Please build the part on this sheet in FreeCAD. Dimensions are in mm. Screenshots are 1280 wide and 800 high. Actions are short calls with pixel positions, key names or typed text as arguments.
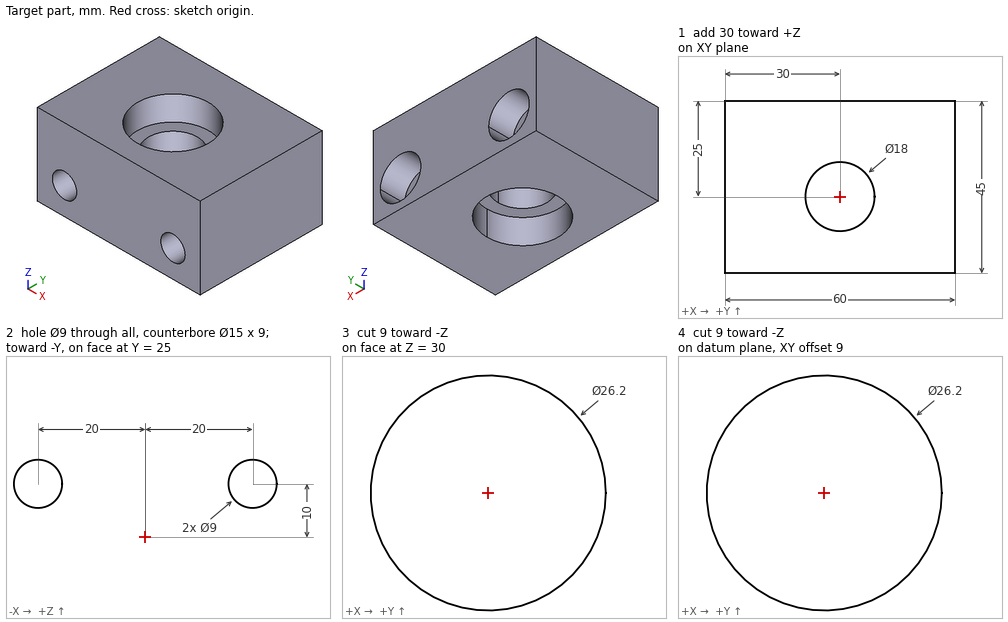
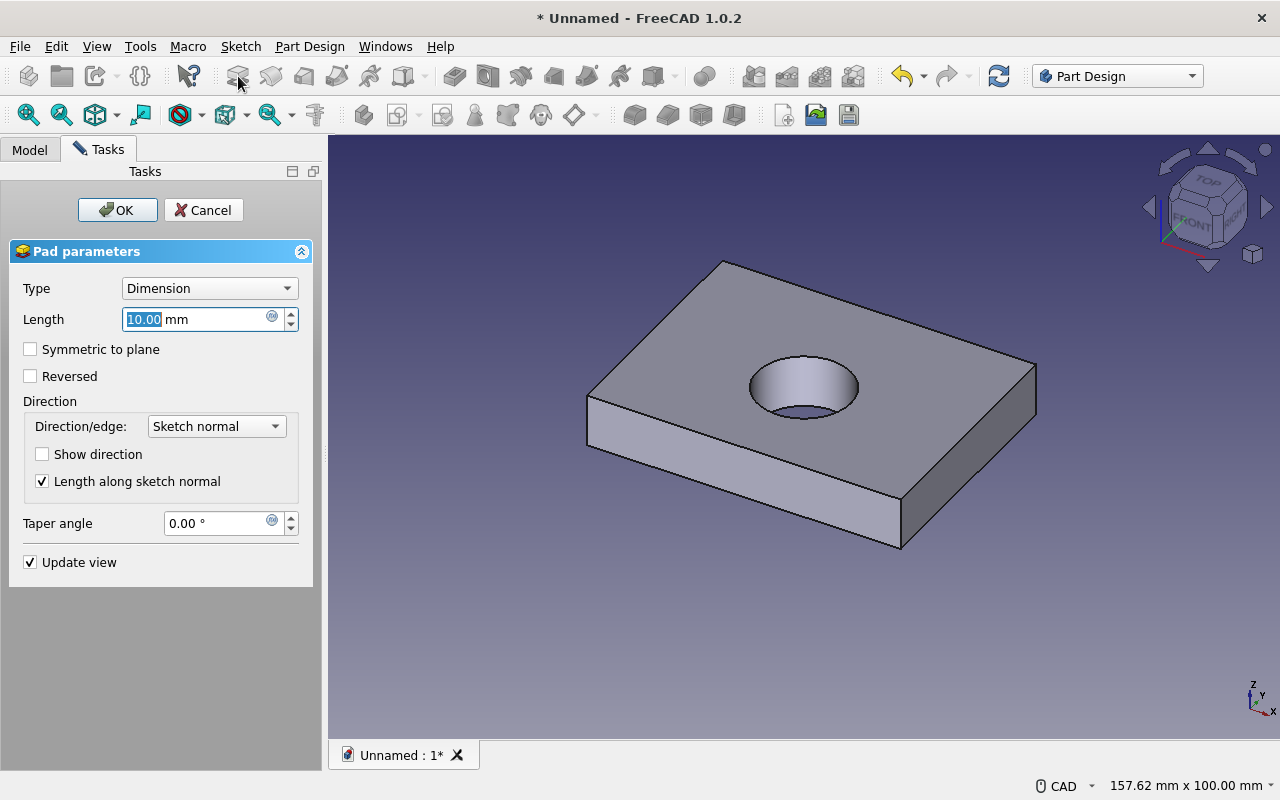
text(30)
key(Tab)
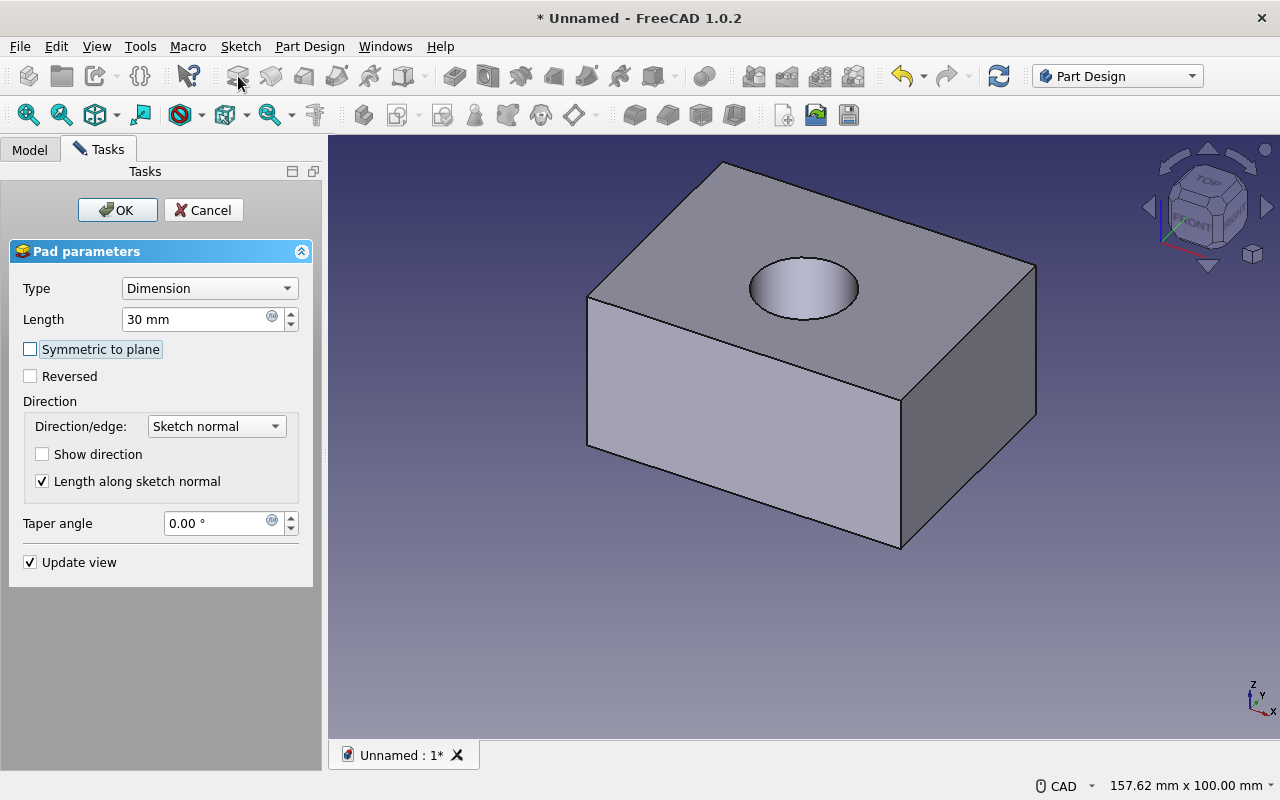
click(118, 210)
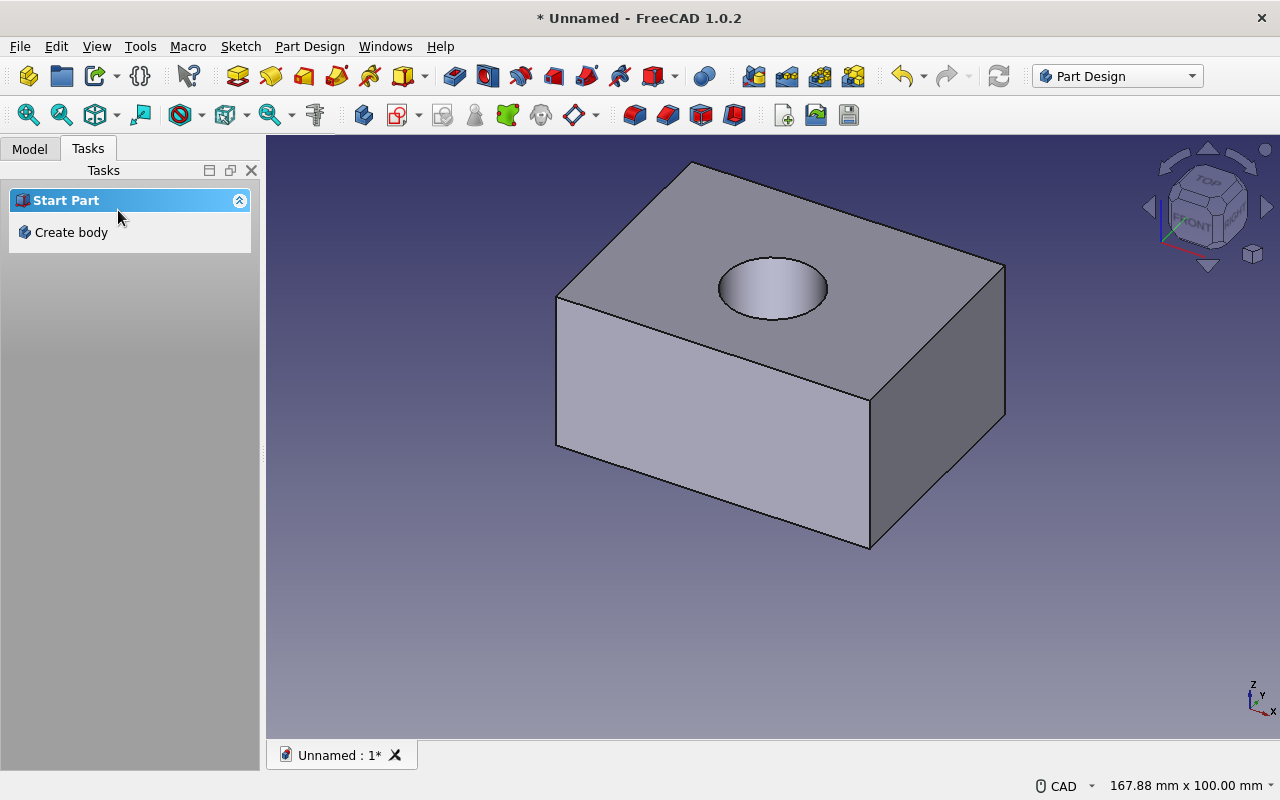
key(4)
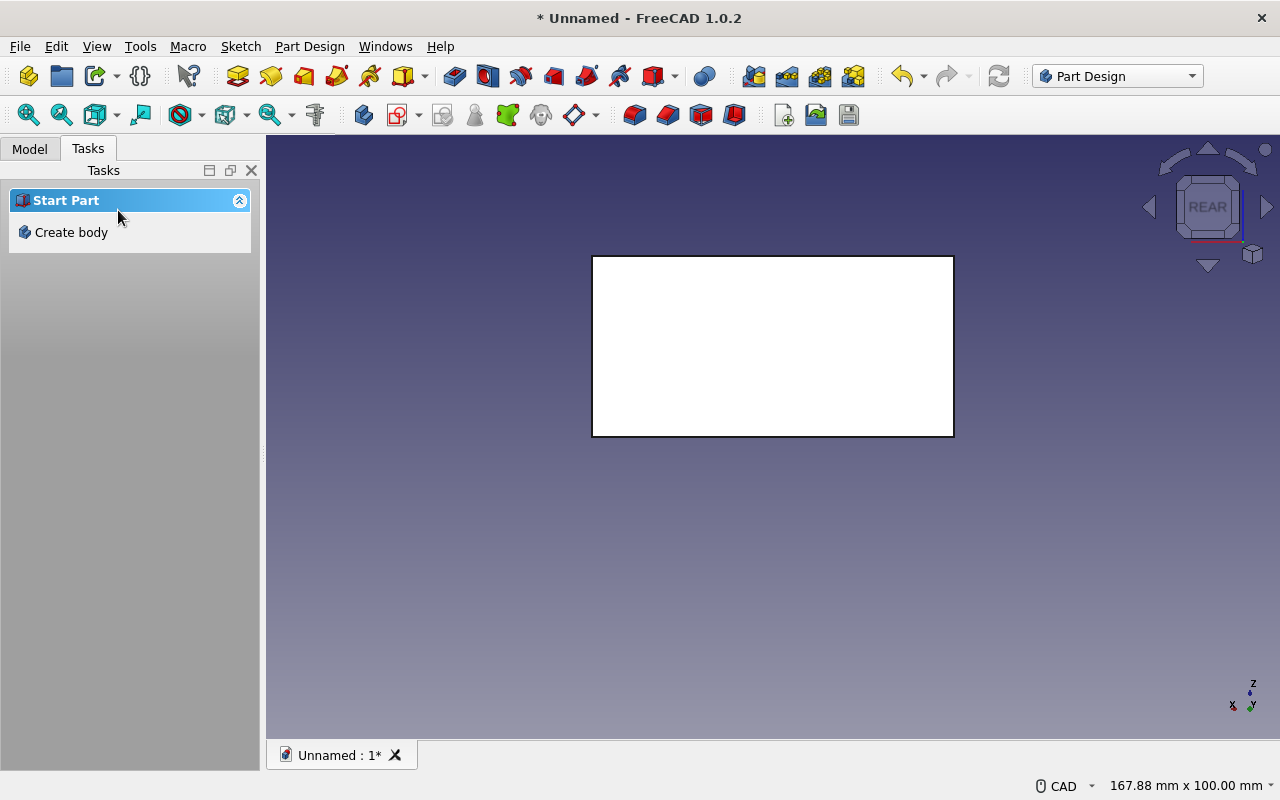
click(29, 116)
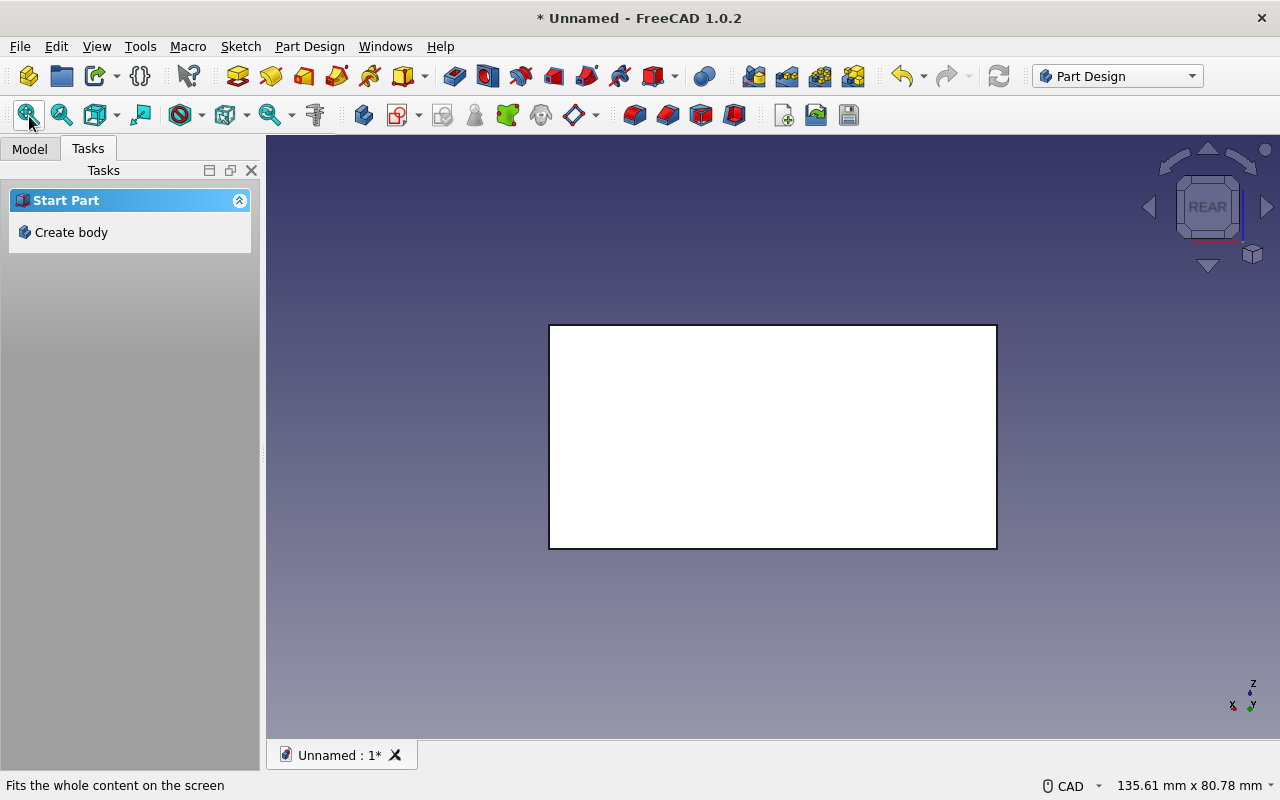
click(709, 436)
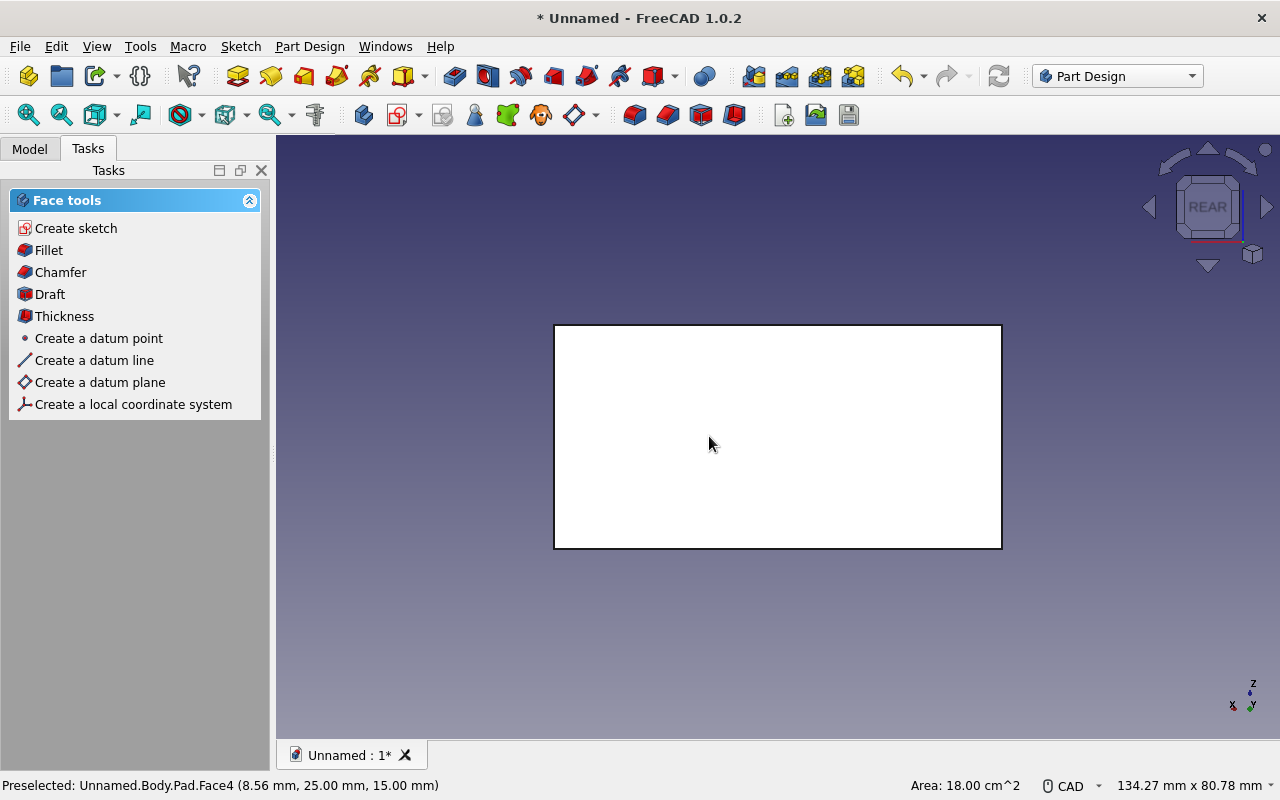
click(396, 116)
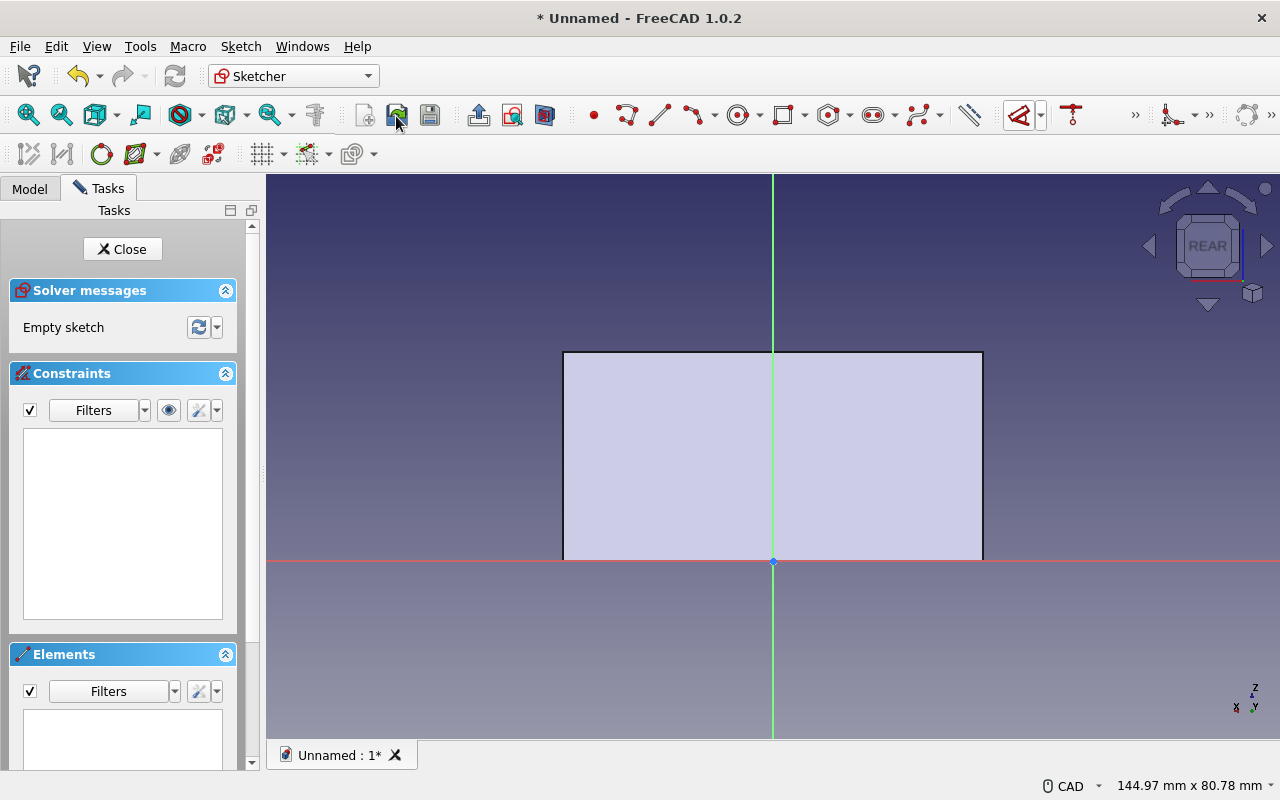
scroll(856, 577, up, 3)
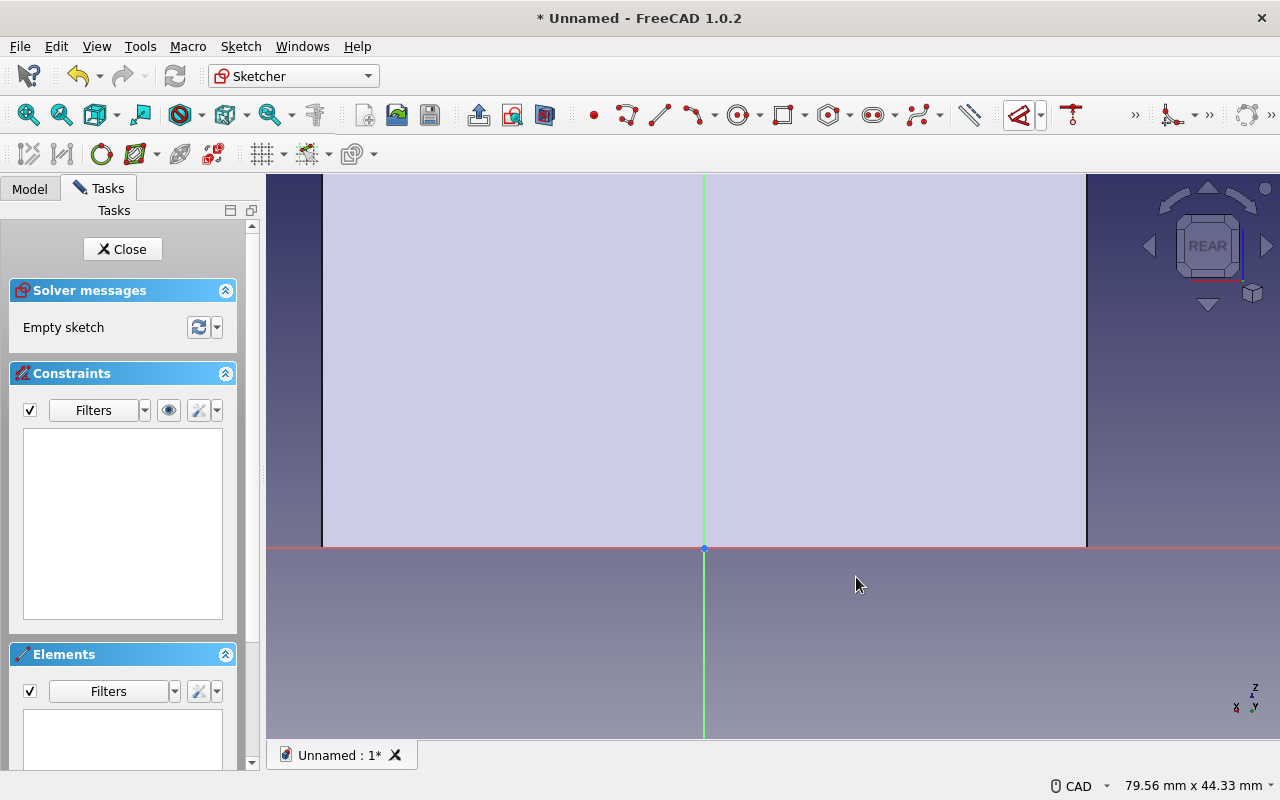
click(738, 116)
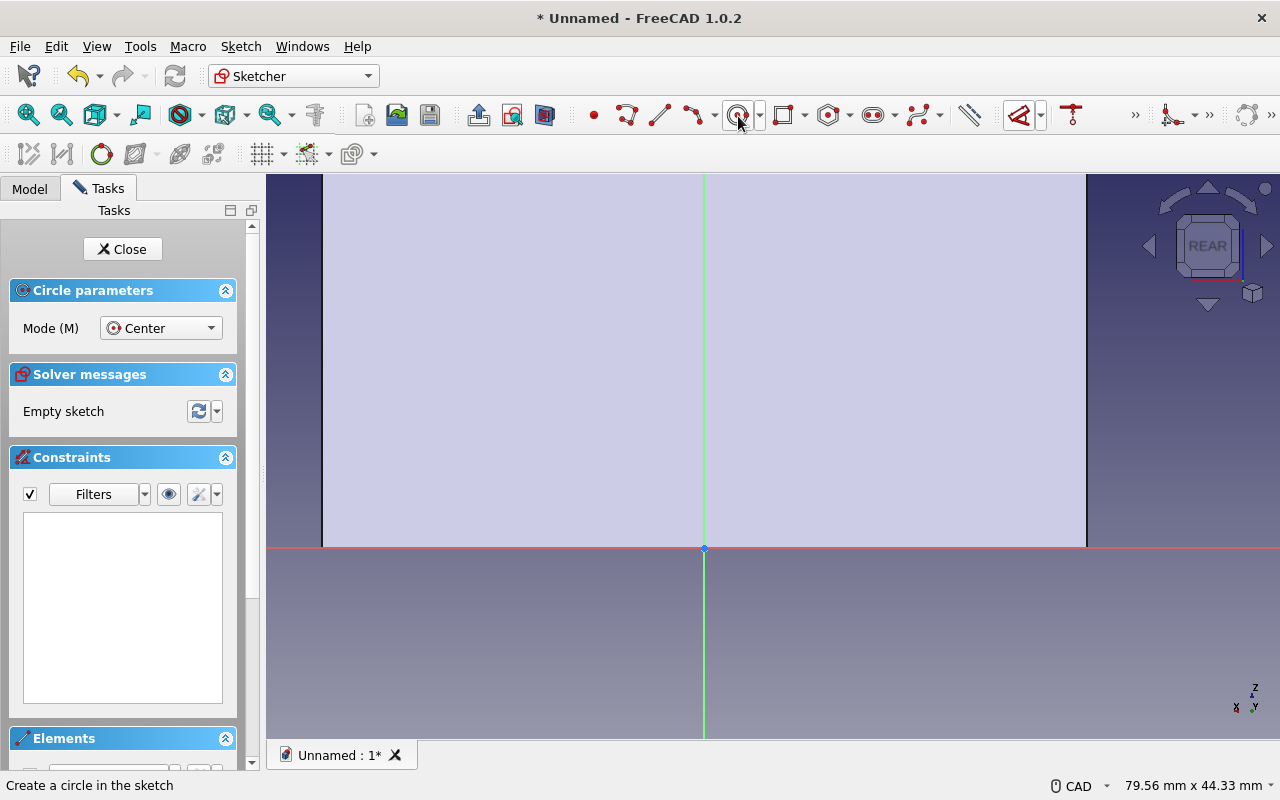
click(959, 421)
move(1000, 380)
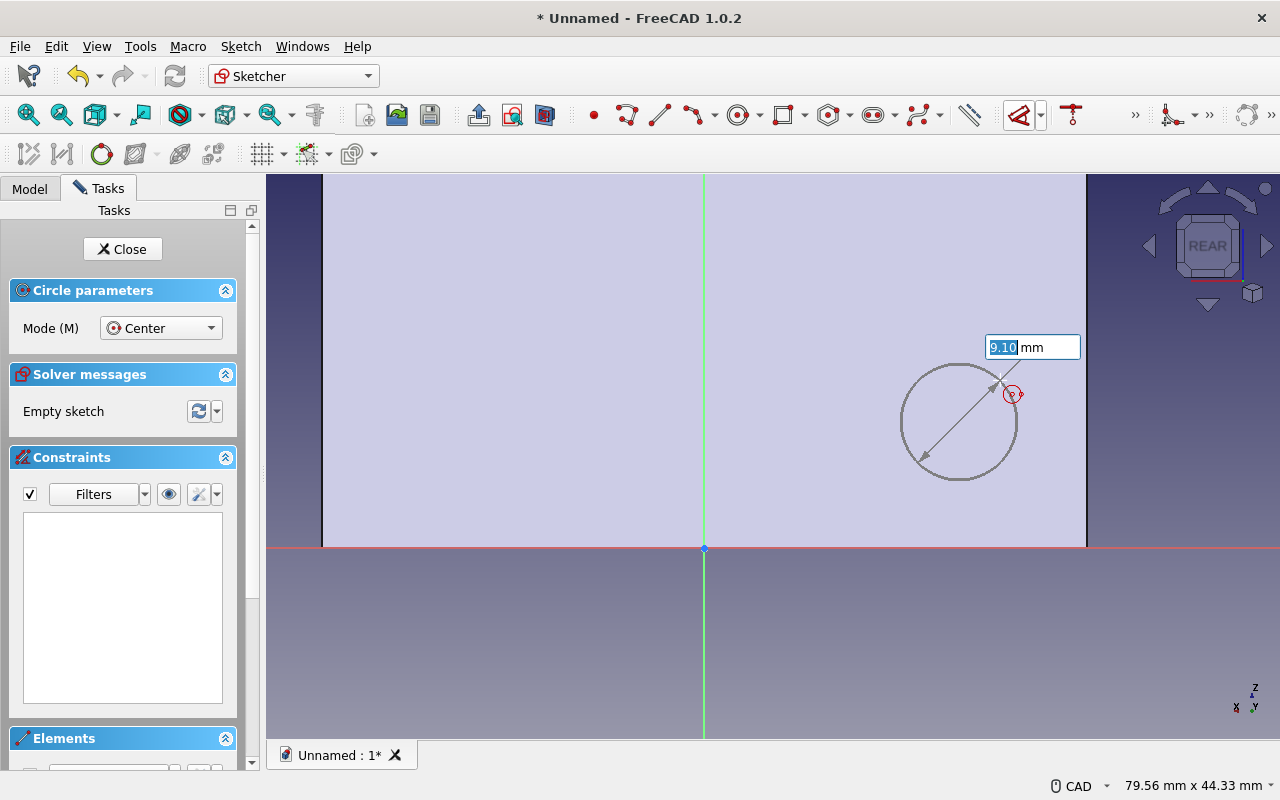
text(9)
key(Return)